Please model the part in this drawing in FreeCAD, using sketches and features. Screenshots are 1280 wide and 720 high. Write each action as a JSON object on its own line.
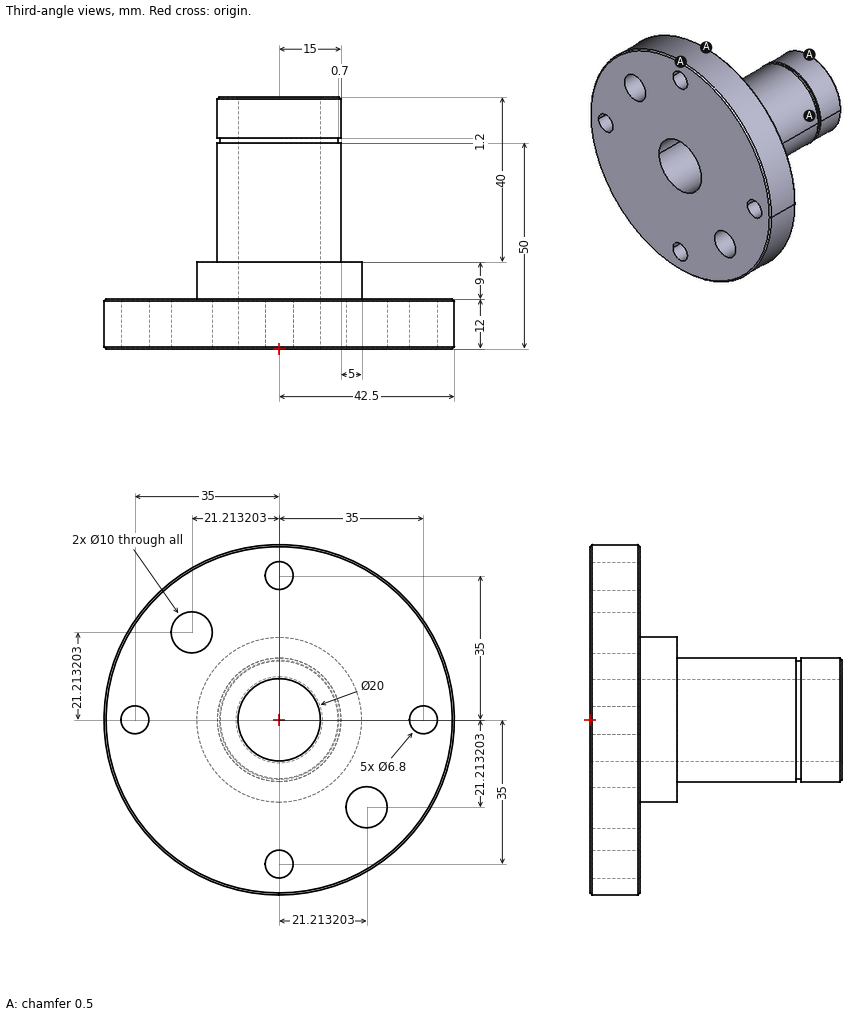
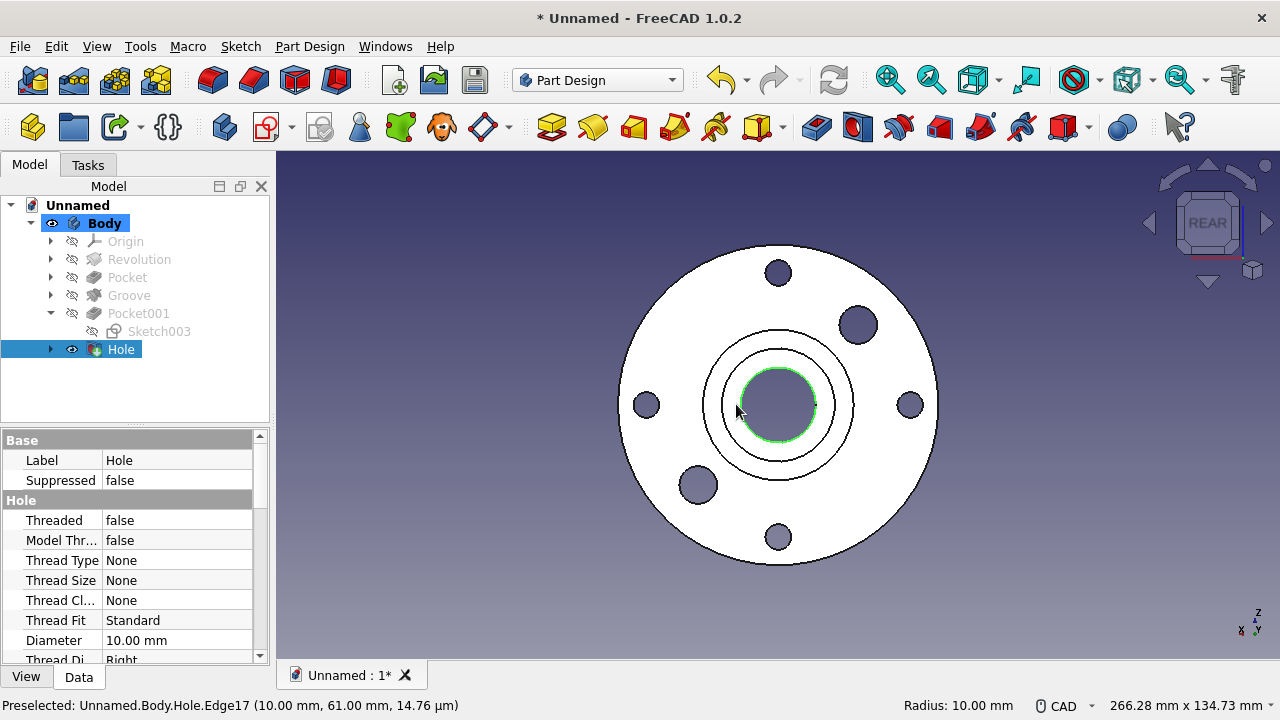
{"action": "left_click", "coordinate": [835, 404], "text": "ctrl"}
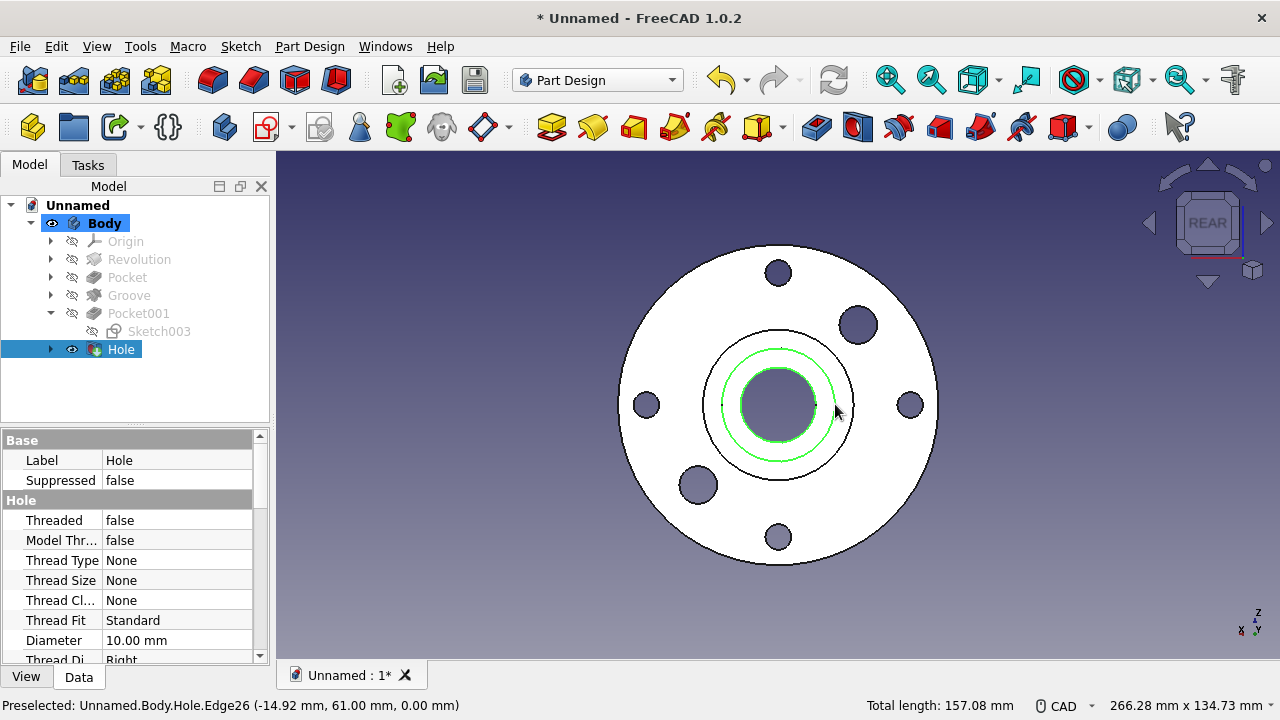
{"action": "left_click", "coordinate": [938, 404], "text": "ctrl"}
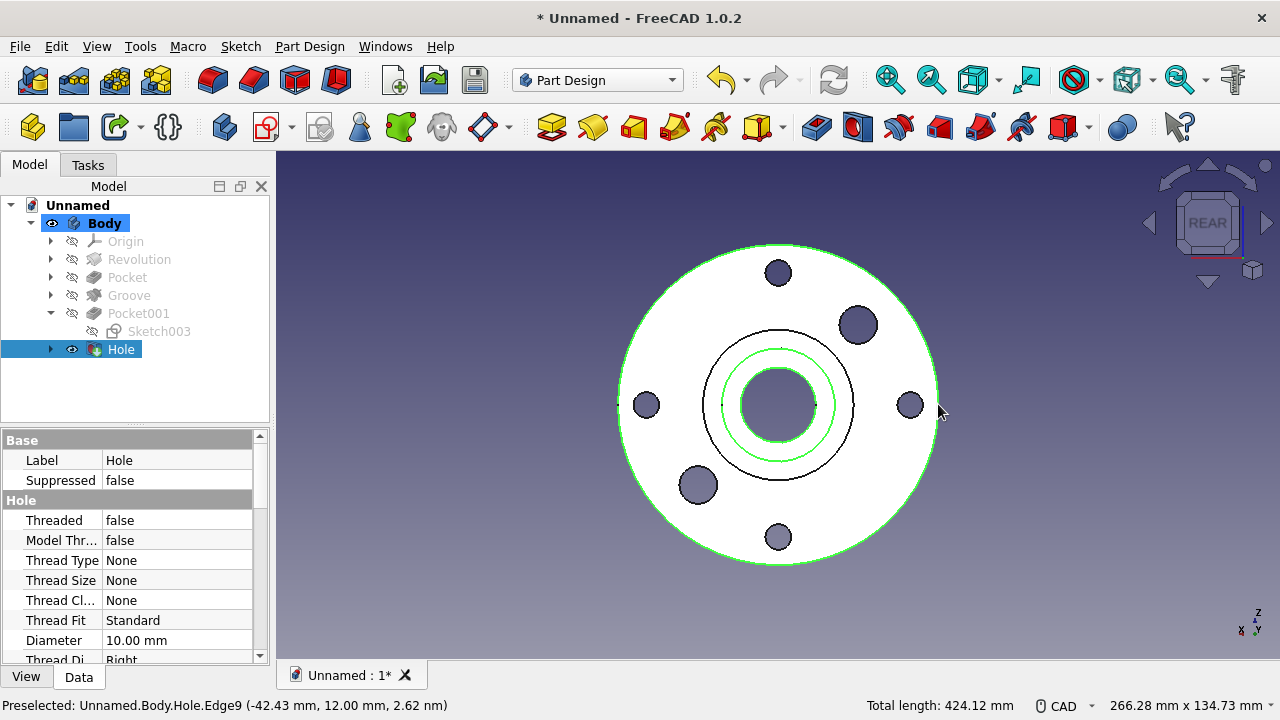
{"action": "key", "text": "0"}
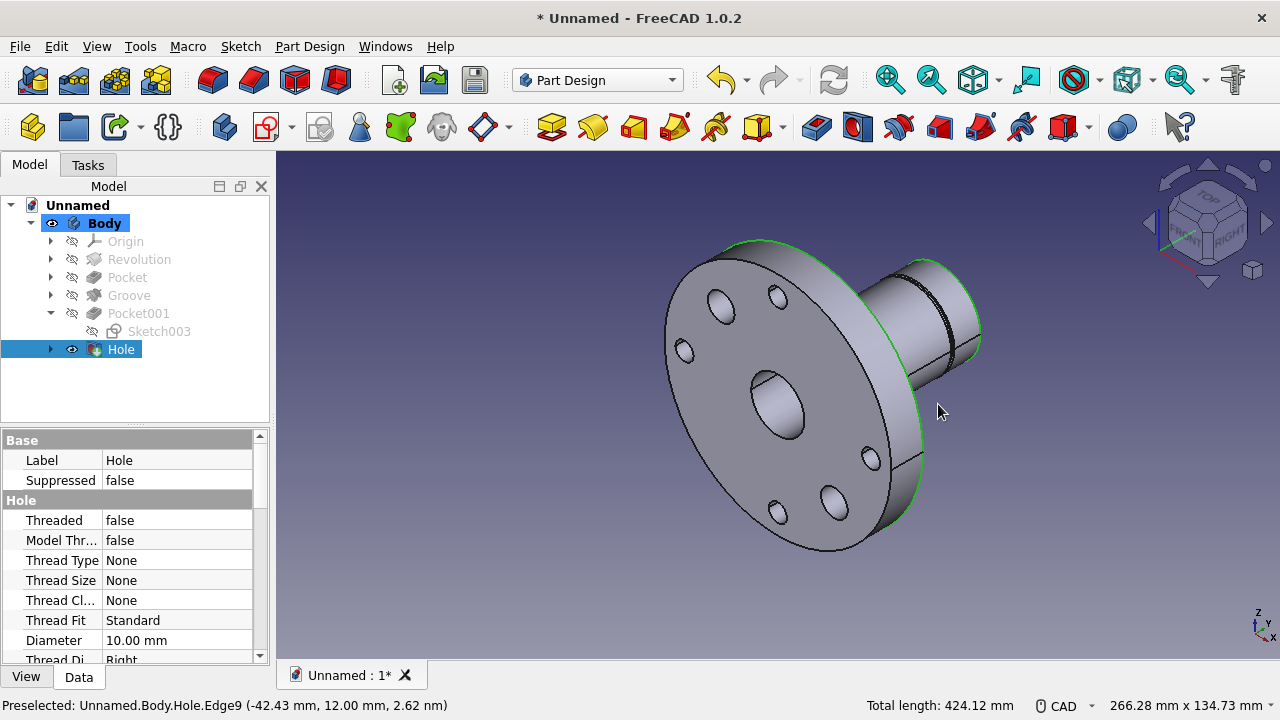
{"action": "key", "text": "v f"}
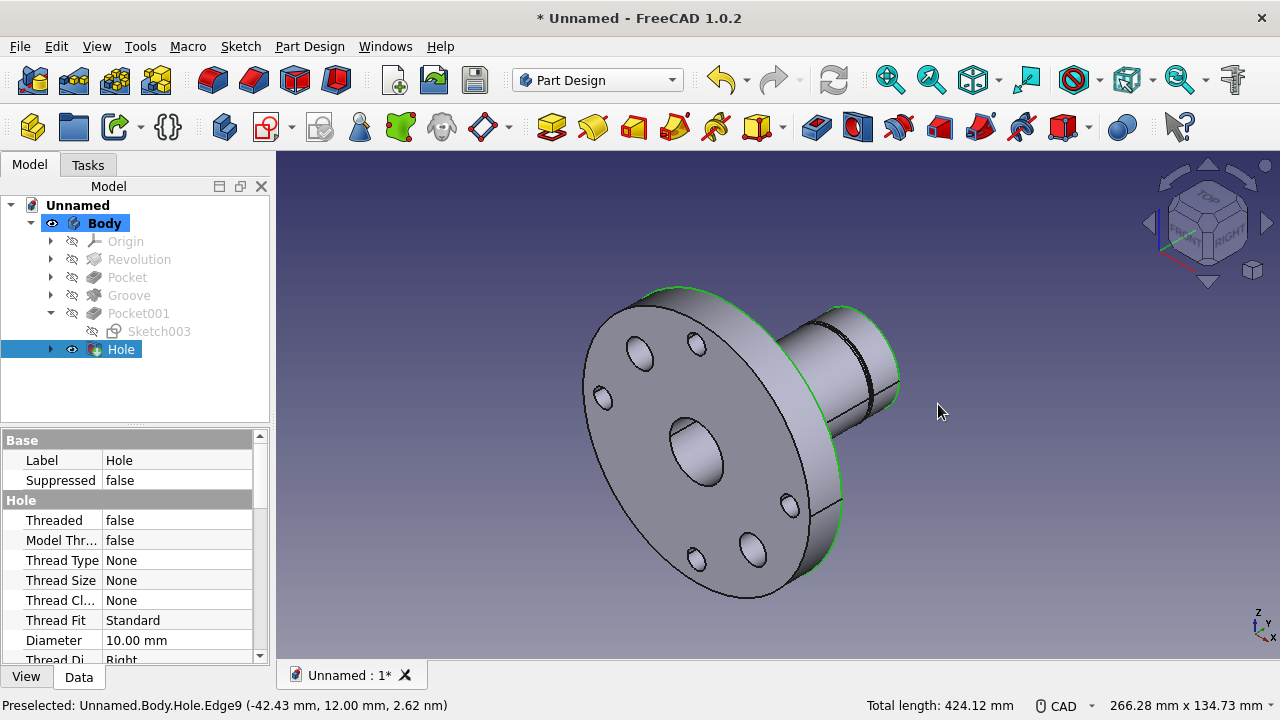
{"action": "left_click", "coordinate": [605, 321], "text": "ctrl"}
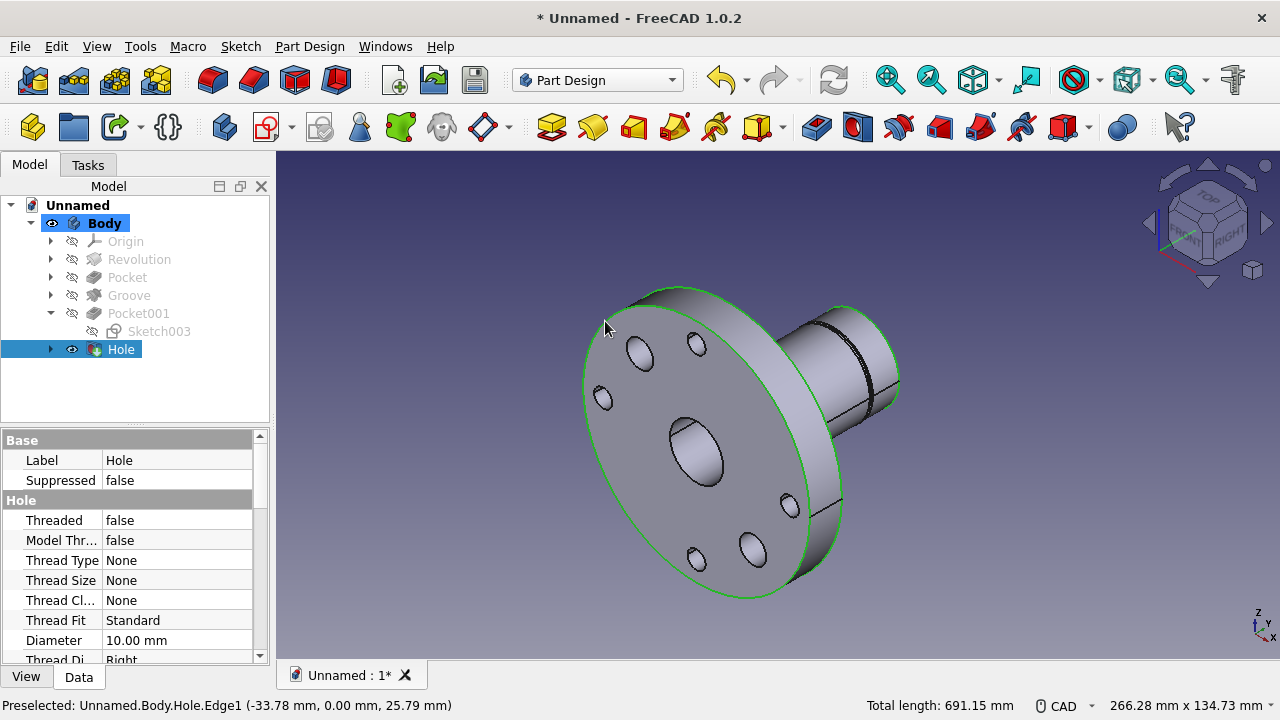
{"action": "left_click", "coordinate": [254, 80]}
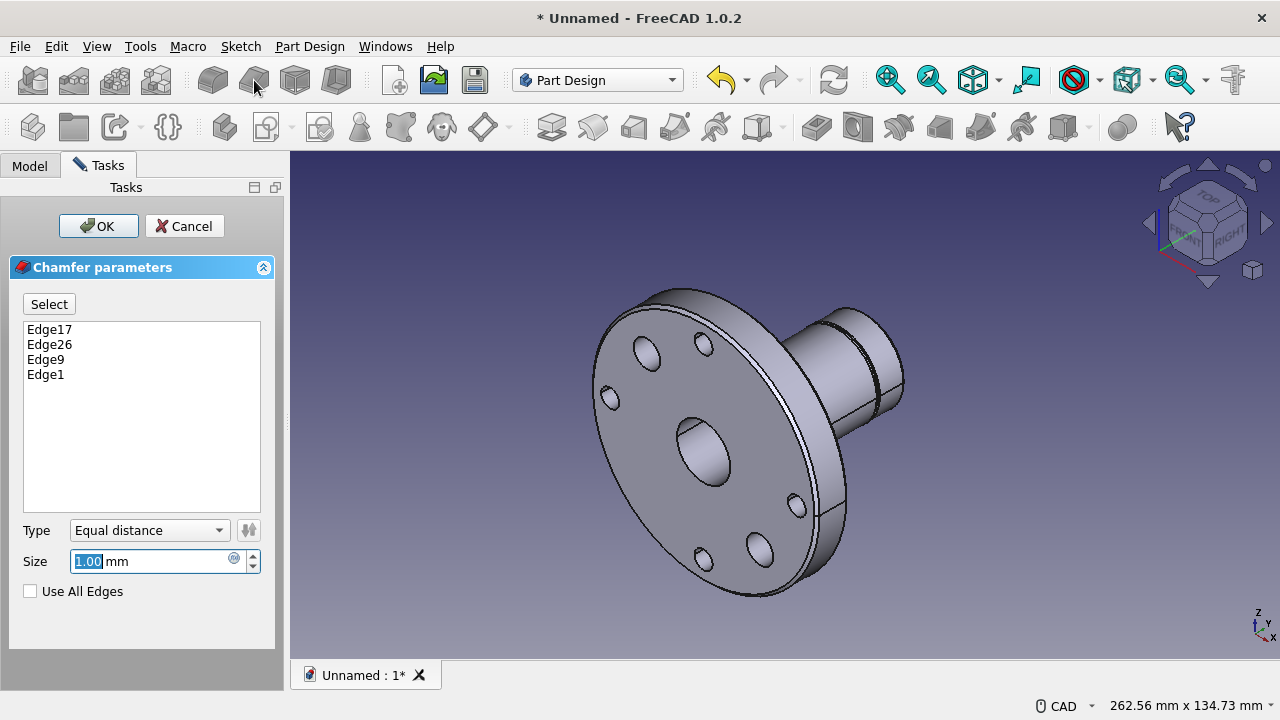
{"action": "type", "text": "0.5"}
{"action": "key", "text": "Tab"}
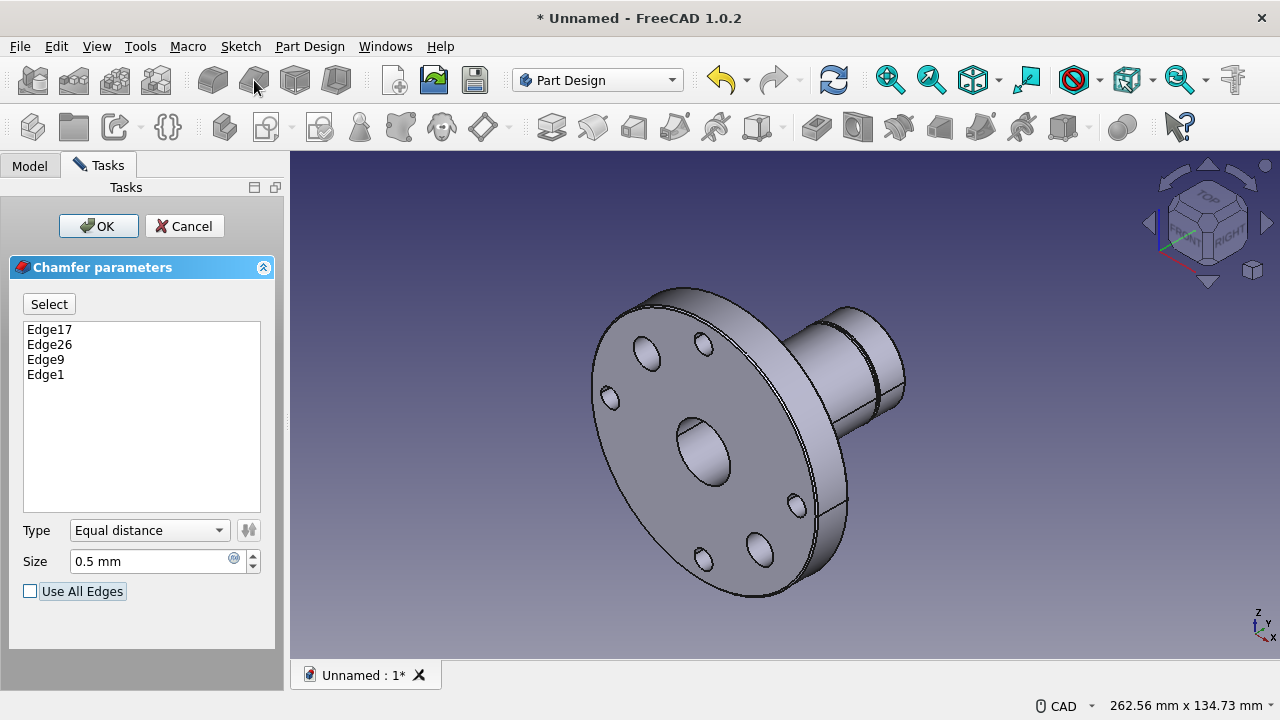
{"action": "left_click", "coordinate": [99, 226]}